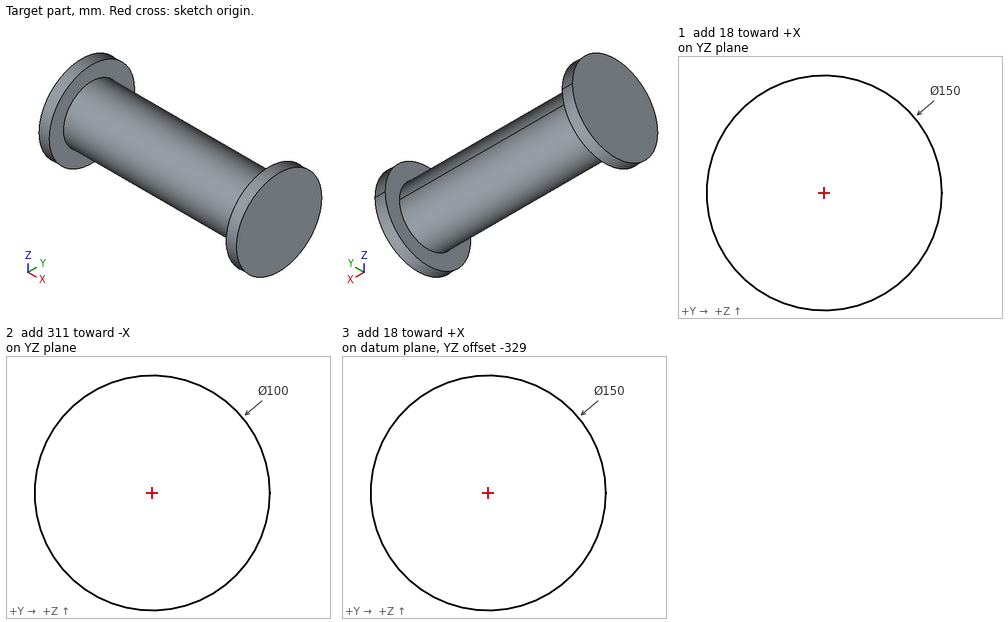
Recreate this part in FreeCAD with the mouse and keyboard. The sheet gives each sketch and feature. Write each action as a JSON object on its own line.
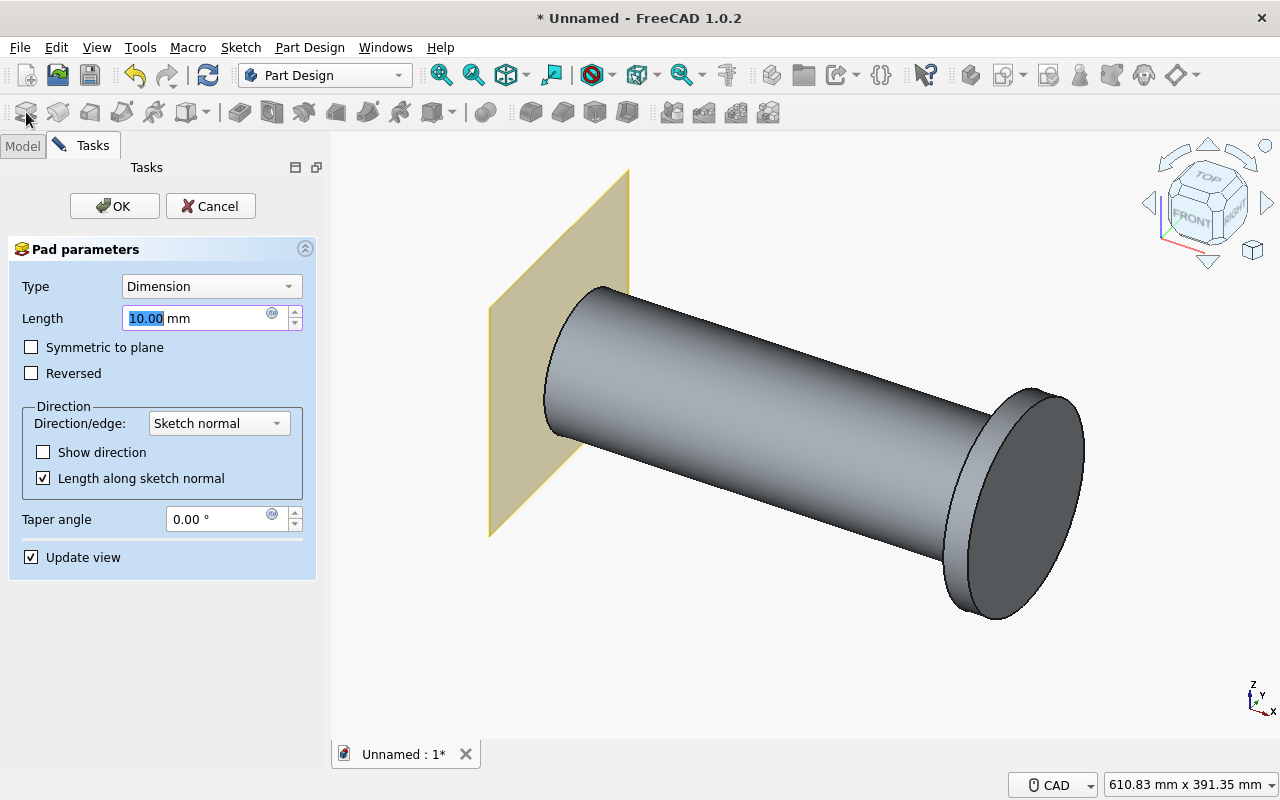
{"action": "type", "text": "18"}
{"action": "key", "text": "Tab"}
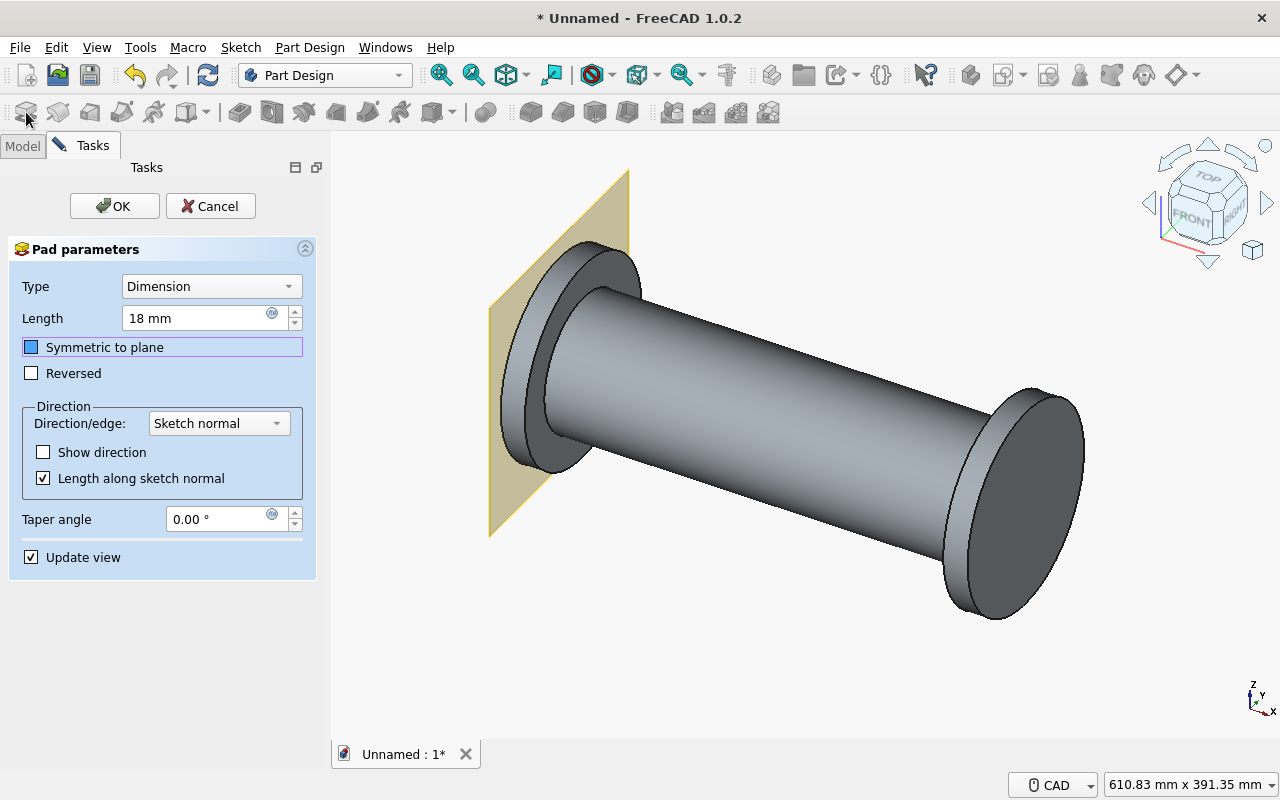
{"action": "left_click", "coordinate": [115, 206]}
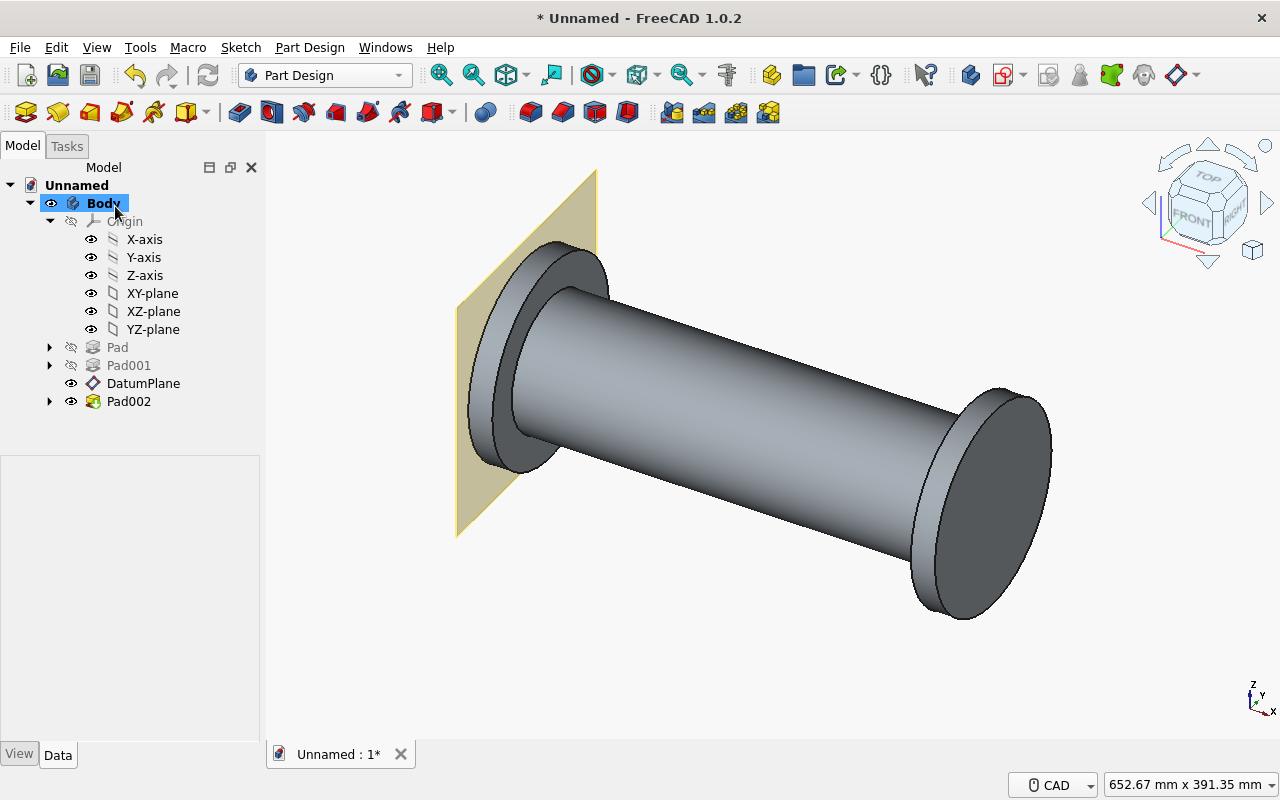
{"action": "left_click", "coordinate": [116, 383]}
{"action": "key", "text": "space"}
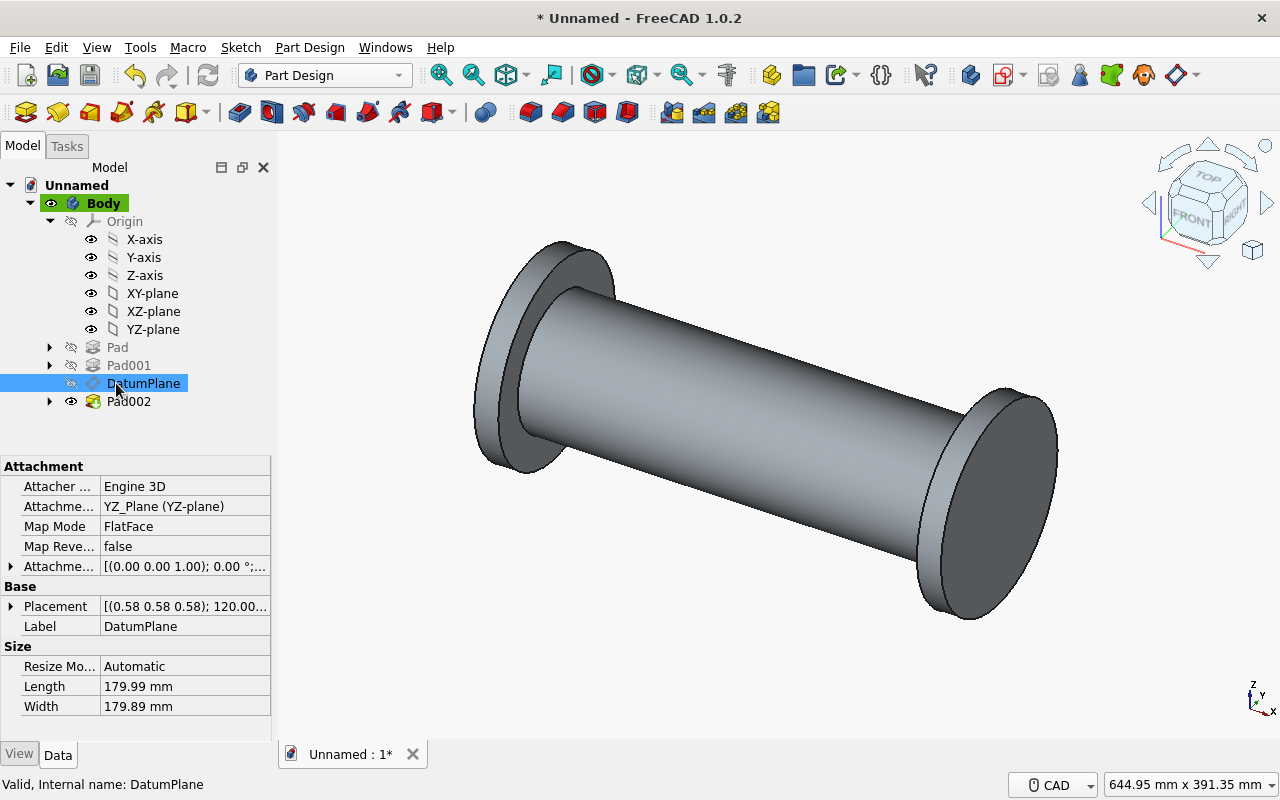
{"action": "key", "text": "0"}